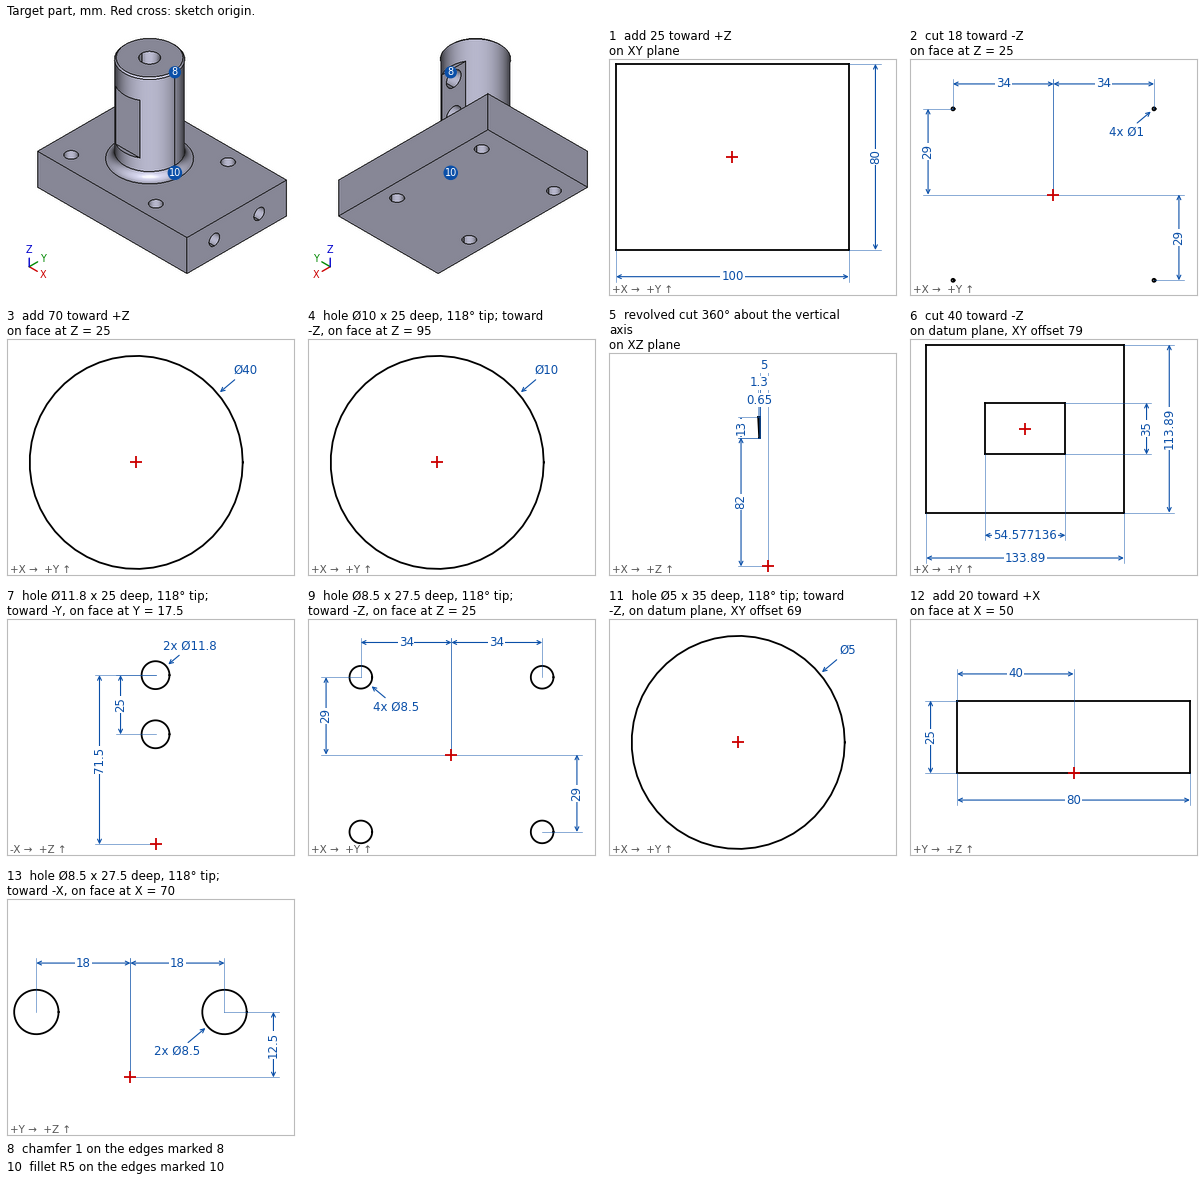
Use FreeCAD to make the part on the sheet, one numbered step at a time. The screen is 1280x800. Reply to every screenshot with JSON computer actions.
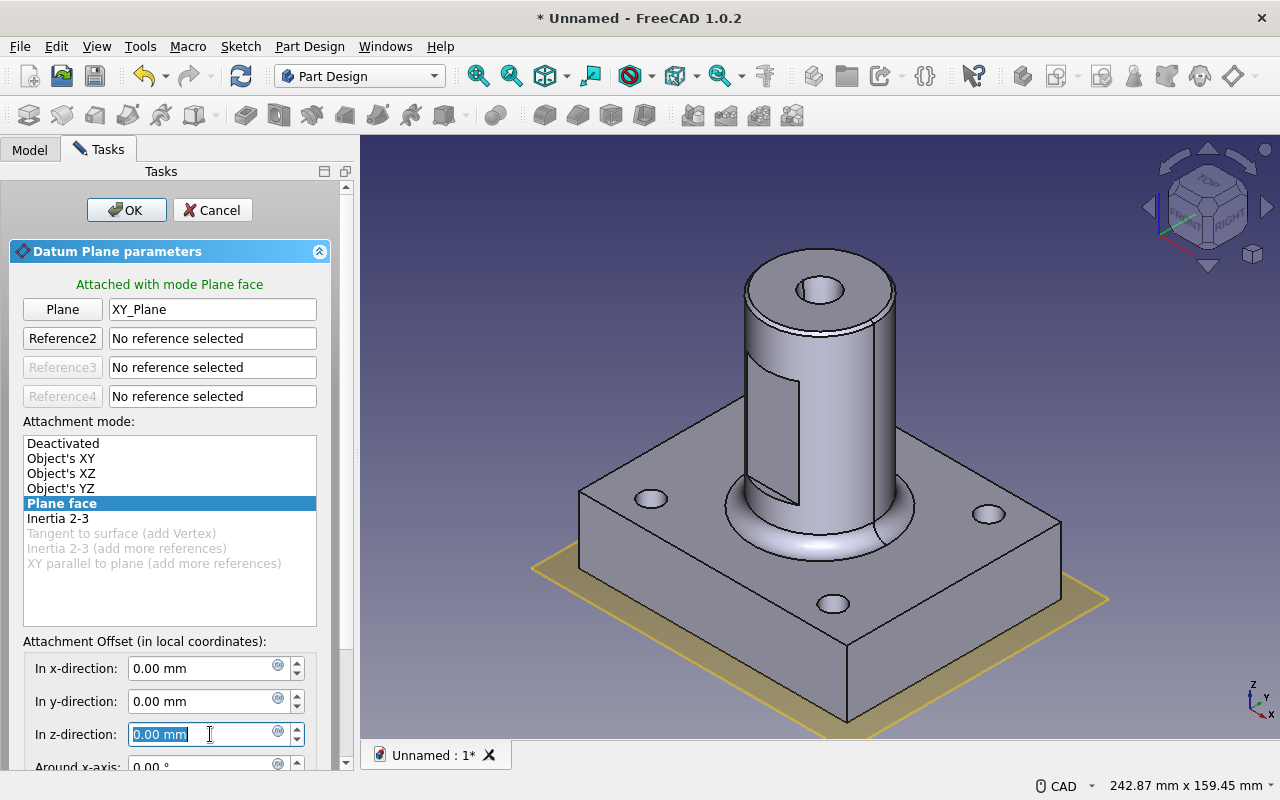
{"action": "type", "text": "69"}
{"action": "key", "text": "Tab"}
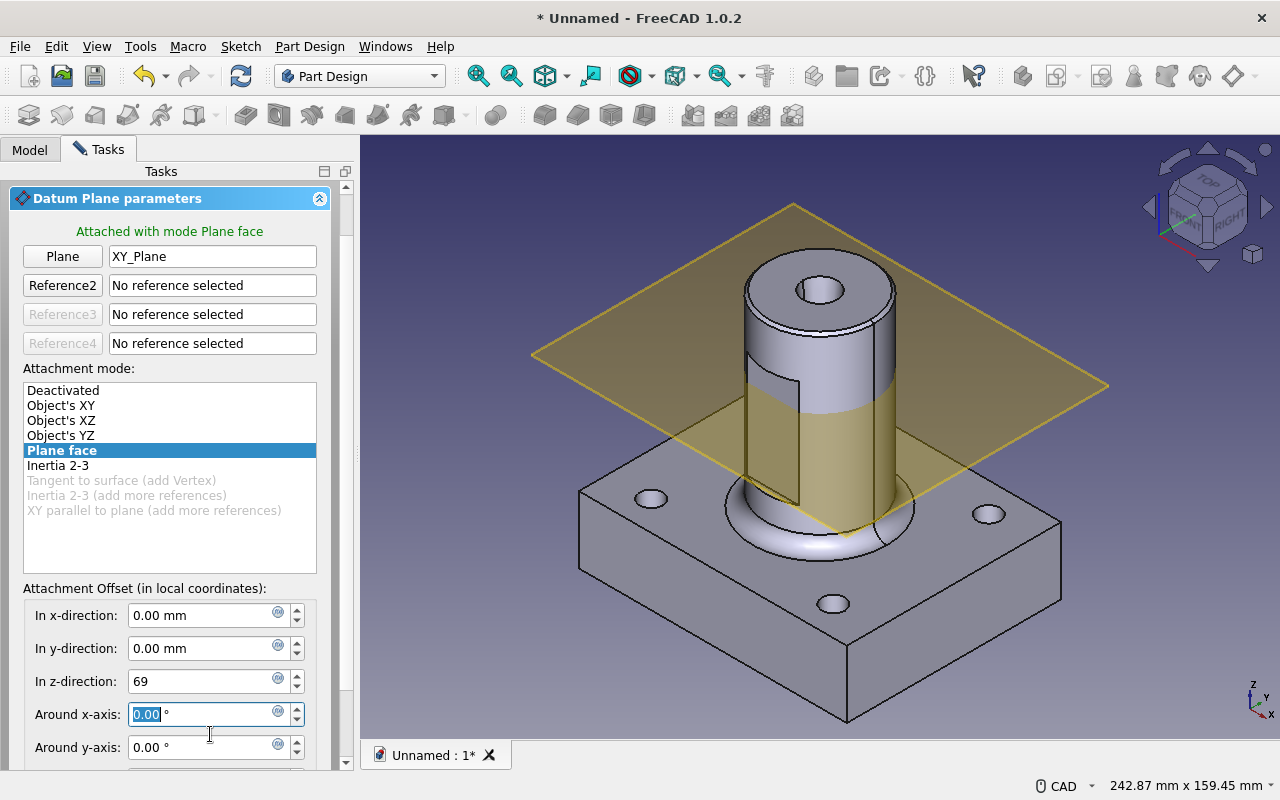
{"action": "scroll", "coordinate": [346, 476], "scroll_direction": "up", "scroll_amount": 2}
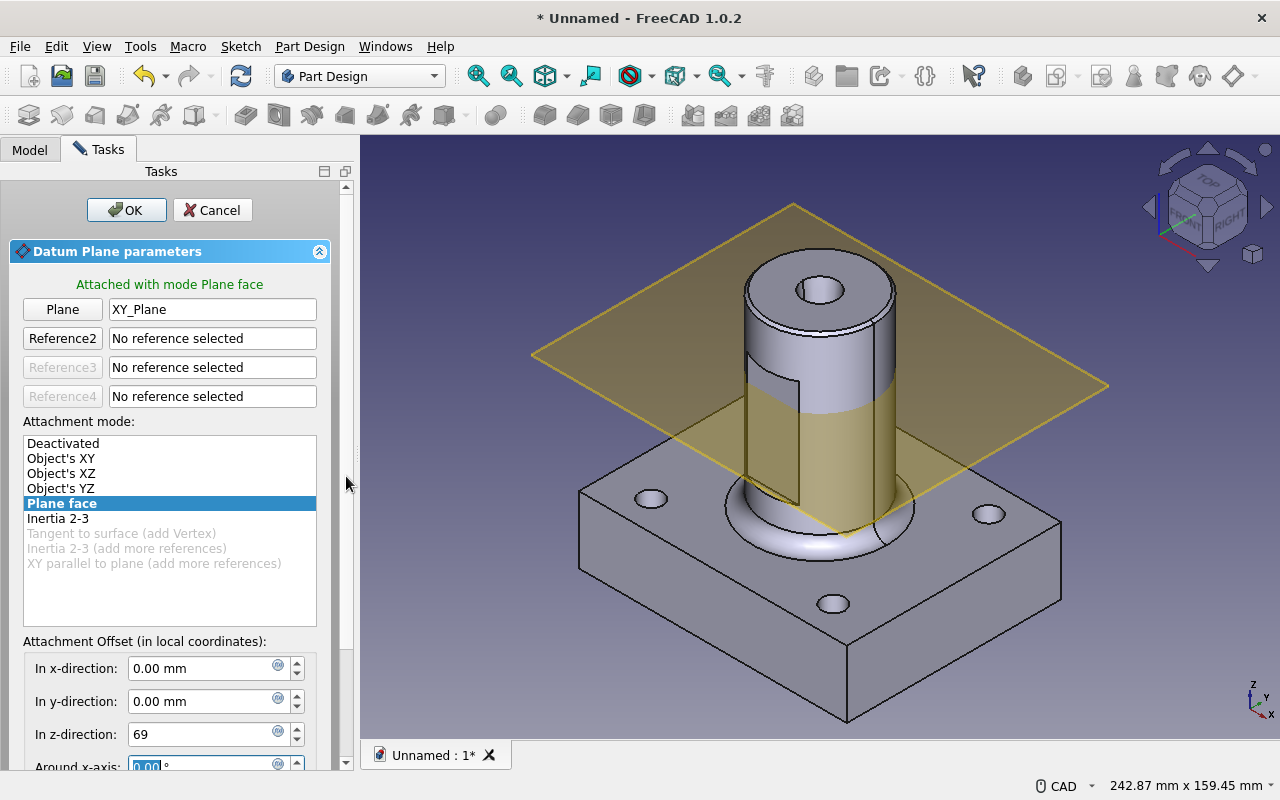
{"action": "left_click", "coordinate": [127, 210]}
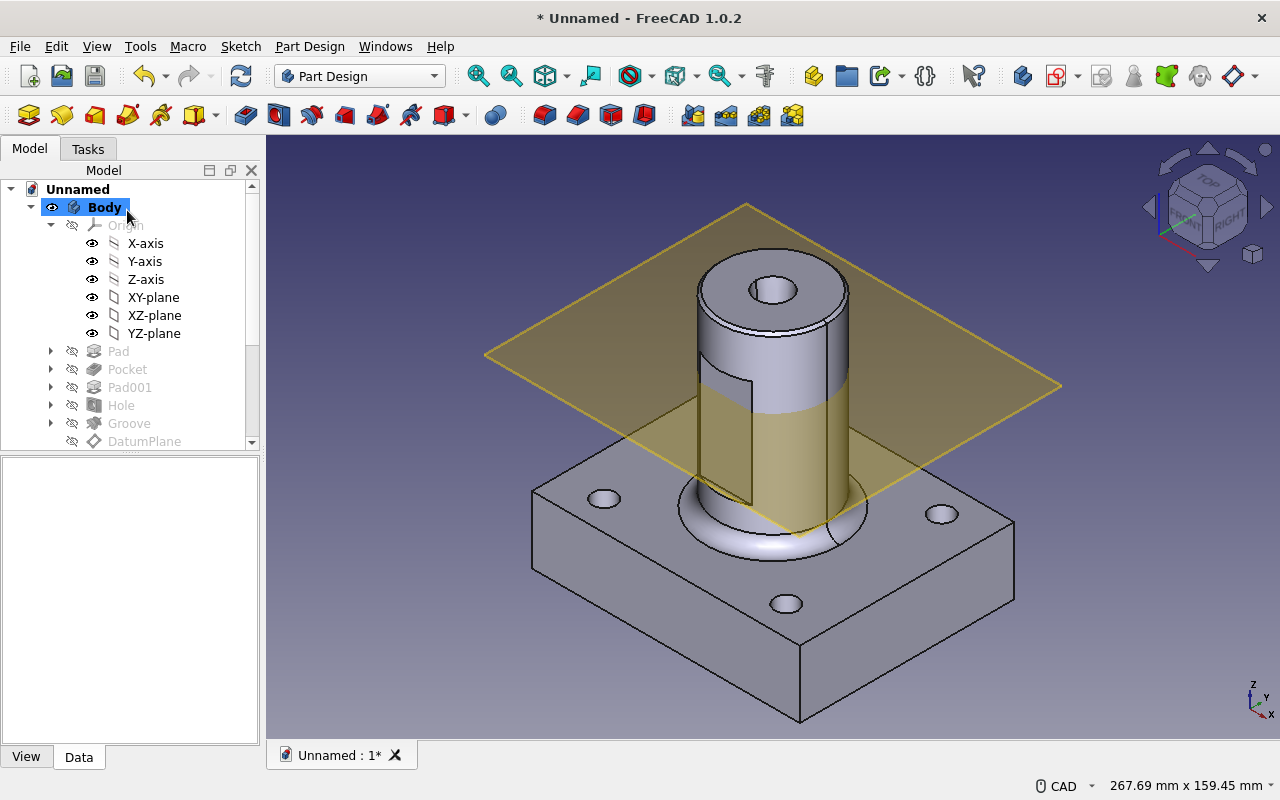
{"action": "scroll", "coordinate": [101, 311], "scroll_direction": "down", "scroll_amount": 3}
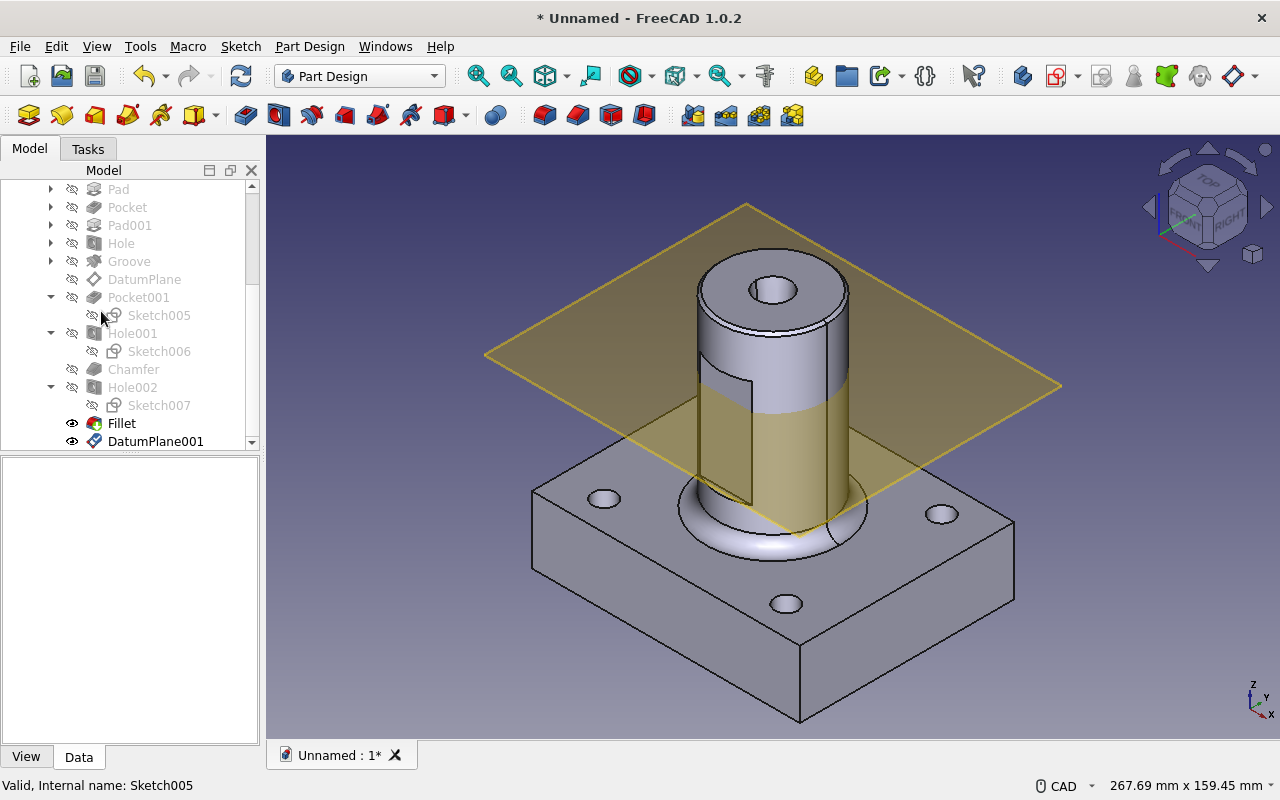
{"action": "left_click", "coordinate": [117, 441]}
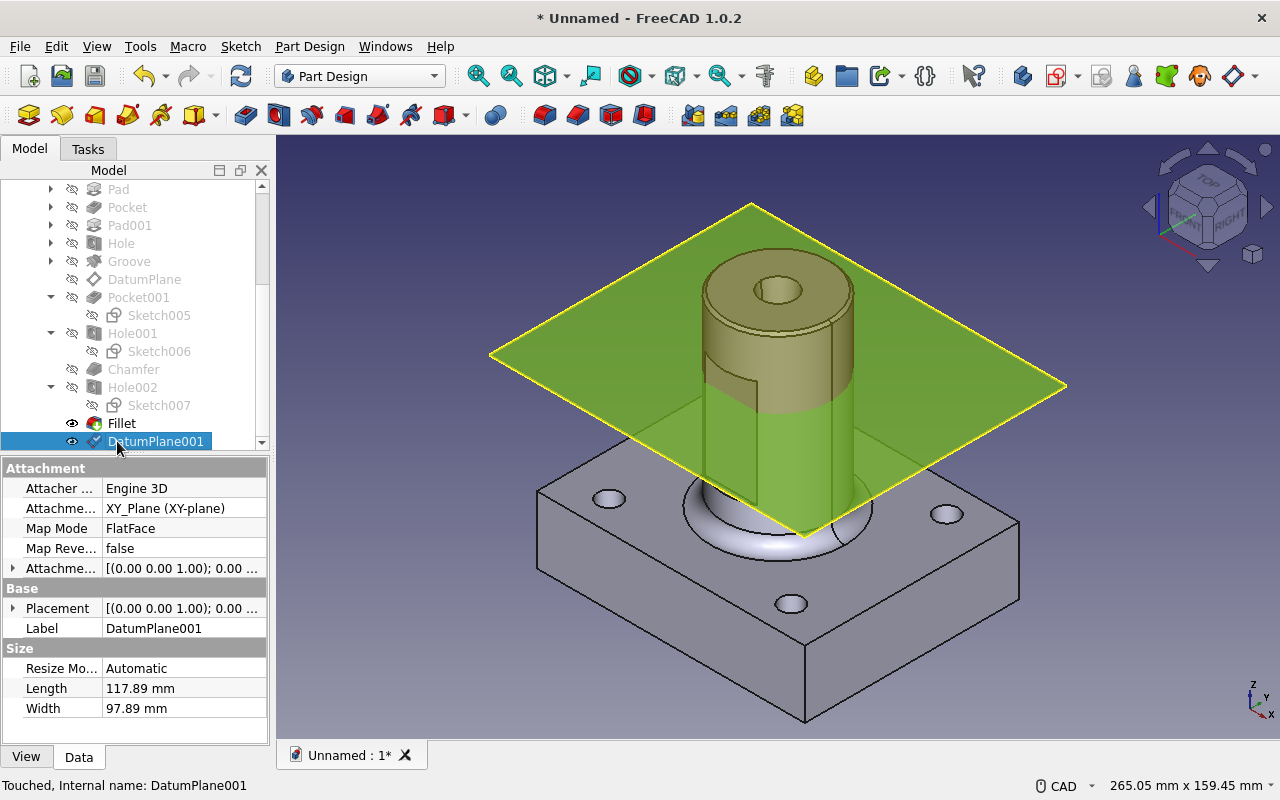
{"action": "left_click", "coordinate": [1056, 76]}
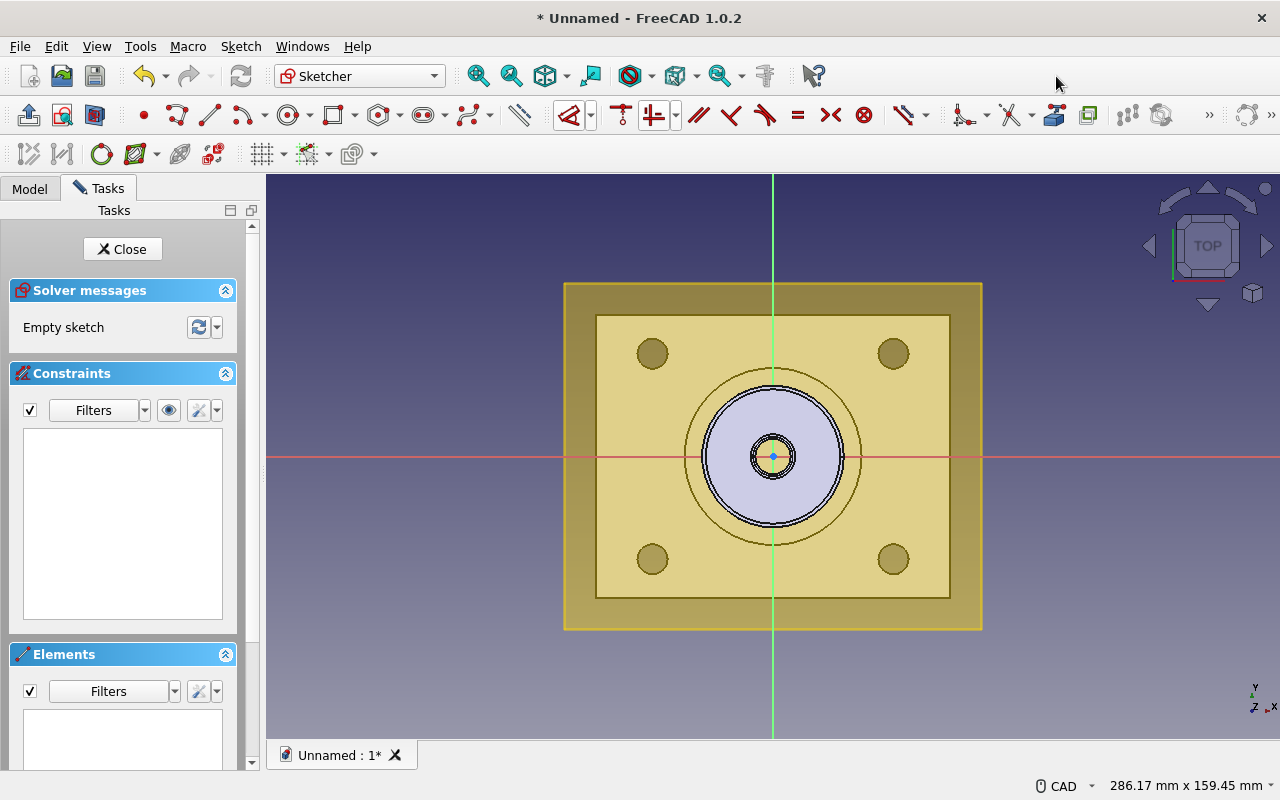
{"action": "left_click", "coordinate": [95, 116]}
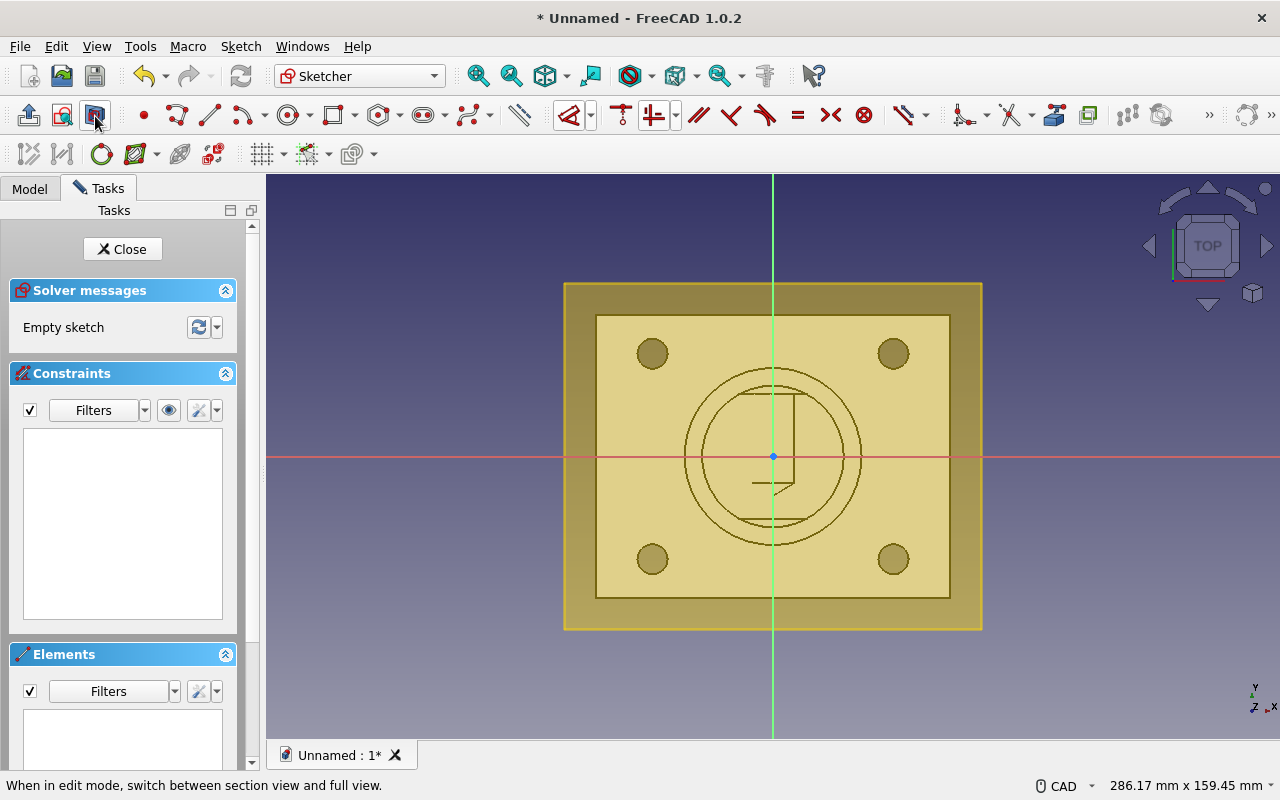
{"action": "scroll", "coordinate": [777, 456], "scroll_direction": "up", "scroll_amount": 15}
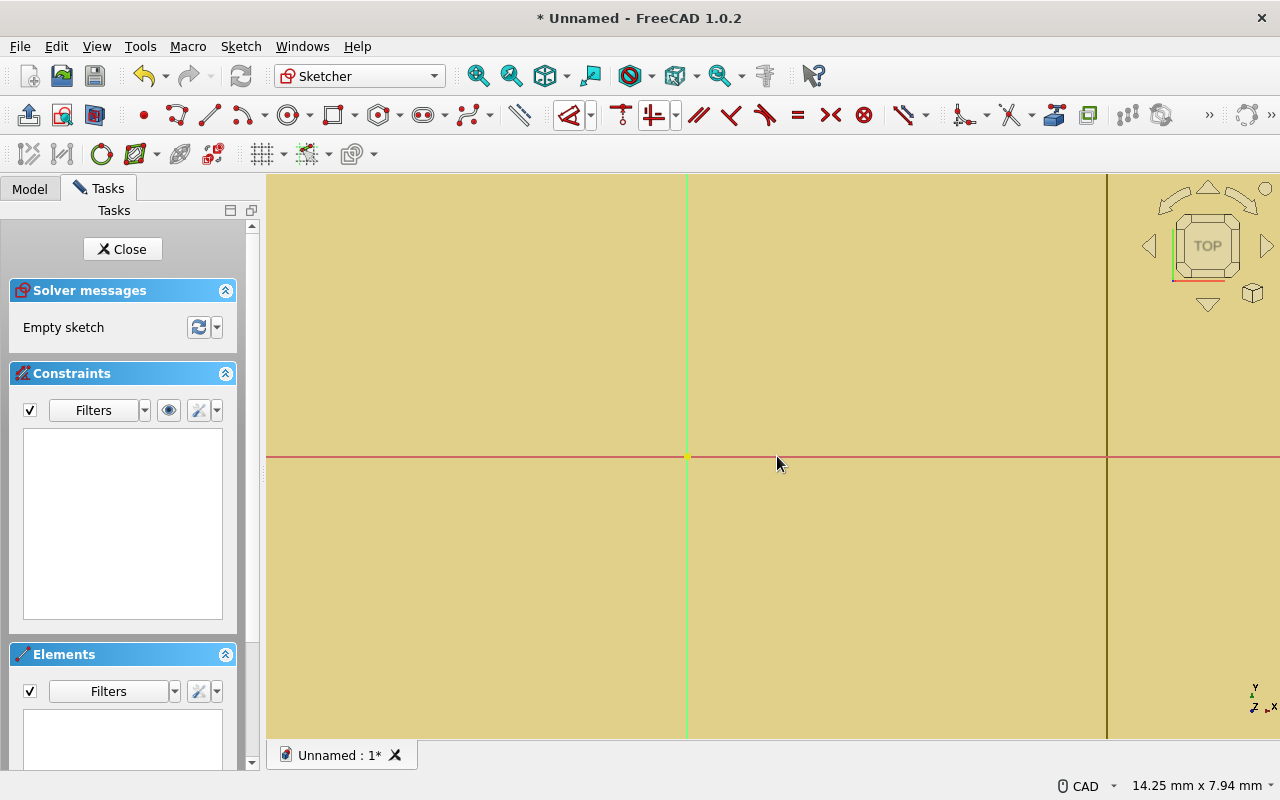
{"action": "key", "text": "g c"}